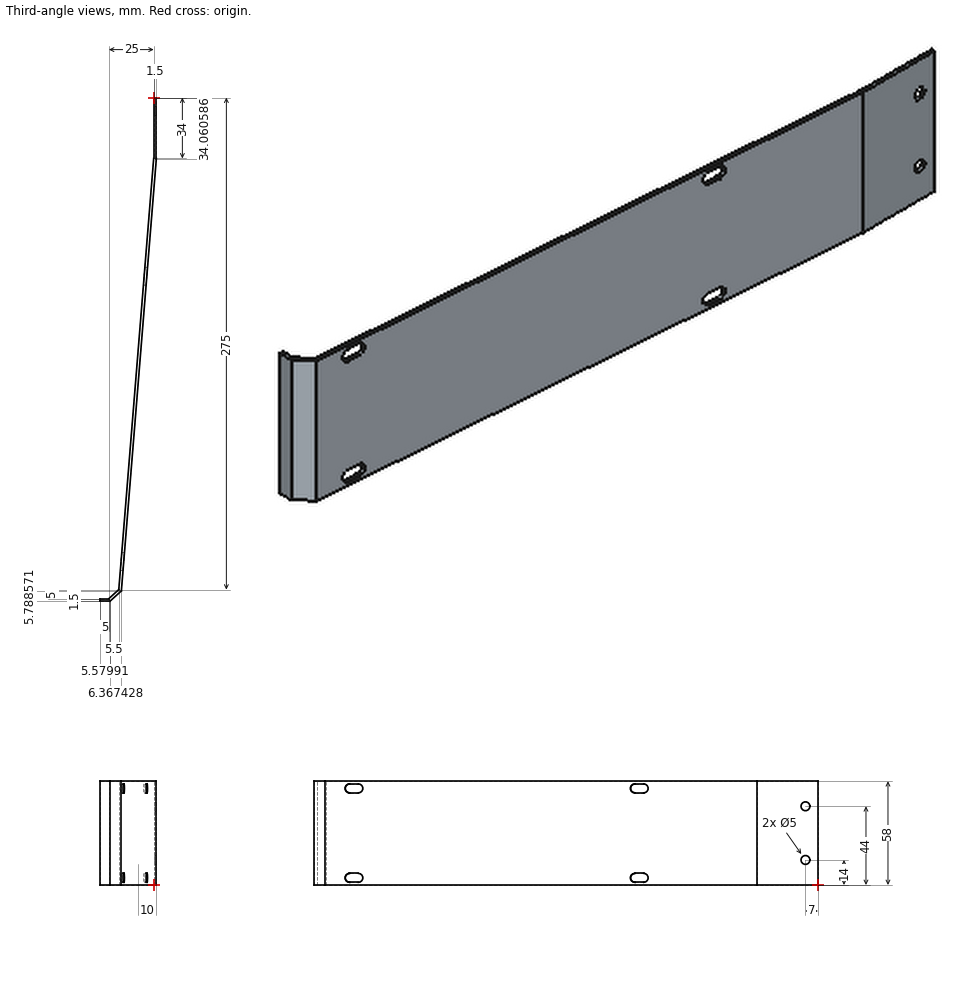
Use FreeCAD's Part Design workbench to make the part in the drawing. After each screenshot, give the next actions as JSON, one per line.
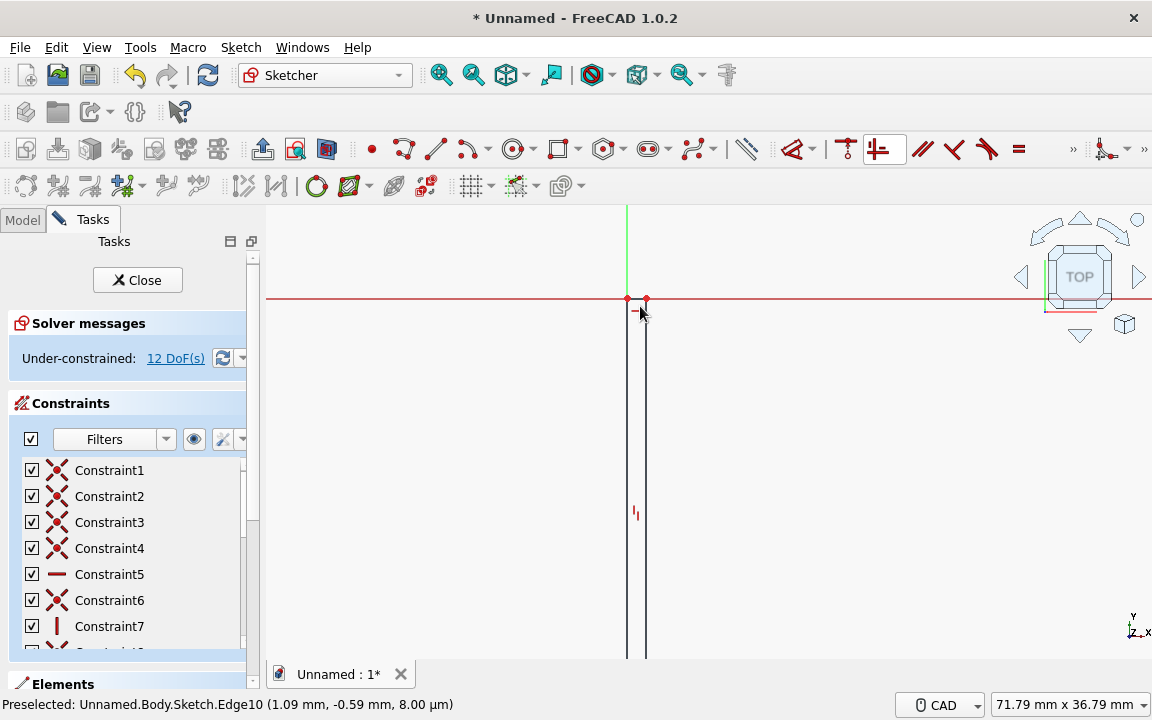
{"action": "left_click", "coordinate": [792, 150]}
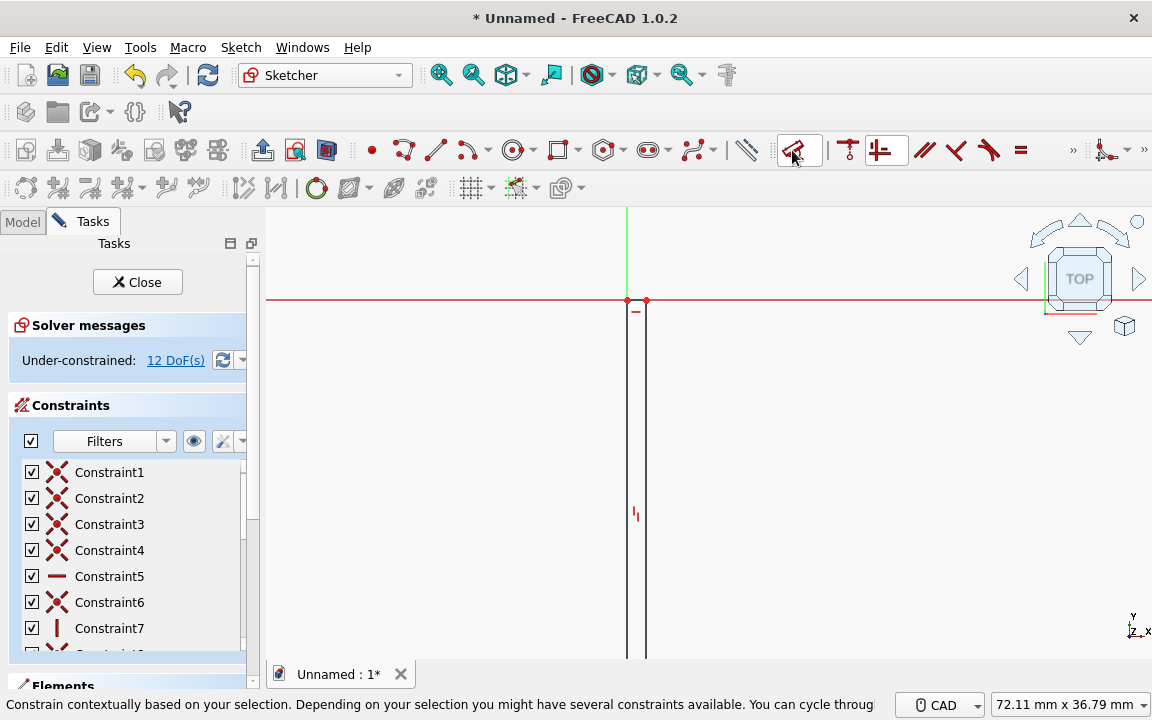
{"action": "scroll", "coordinate": [656, 305], "scroll_direction": "down", "scroll_amount": 13}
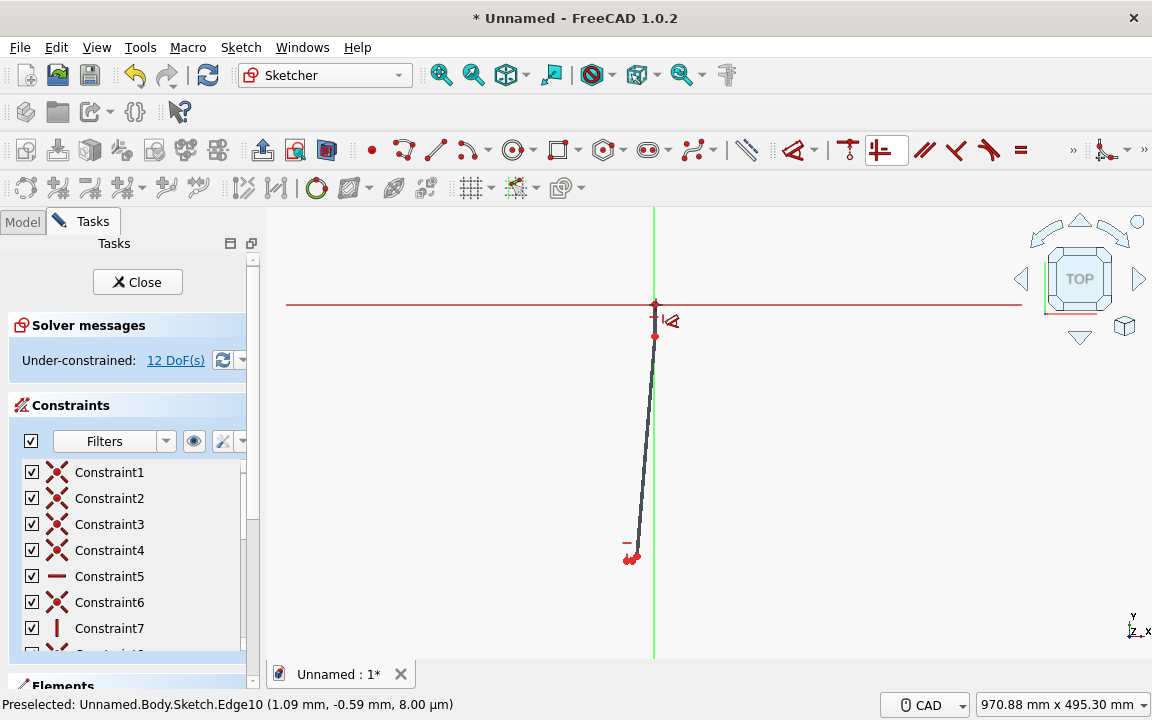
{"action": "scroll", "coordinate": [630, 561], "scroll_direction": "up", "scroll_amount": 13}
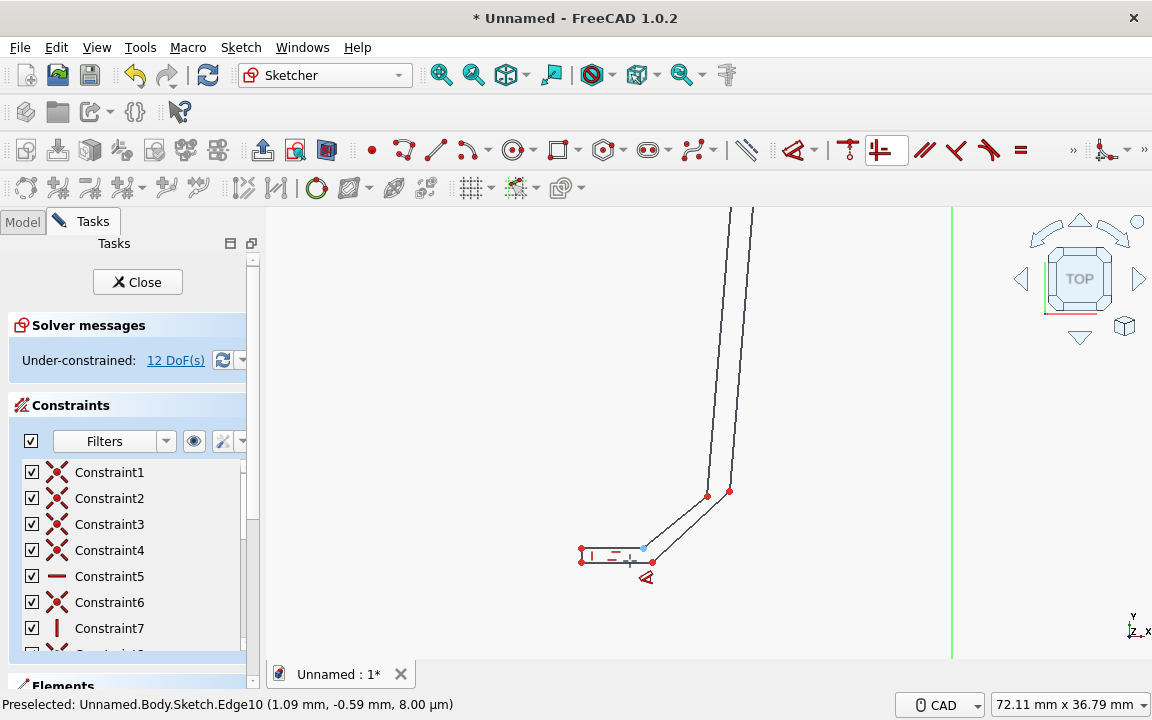
{"action": "left_click", "coordinate": [625, 548]}
{"action": "left_click", "coordinate": [613, 582]}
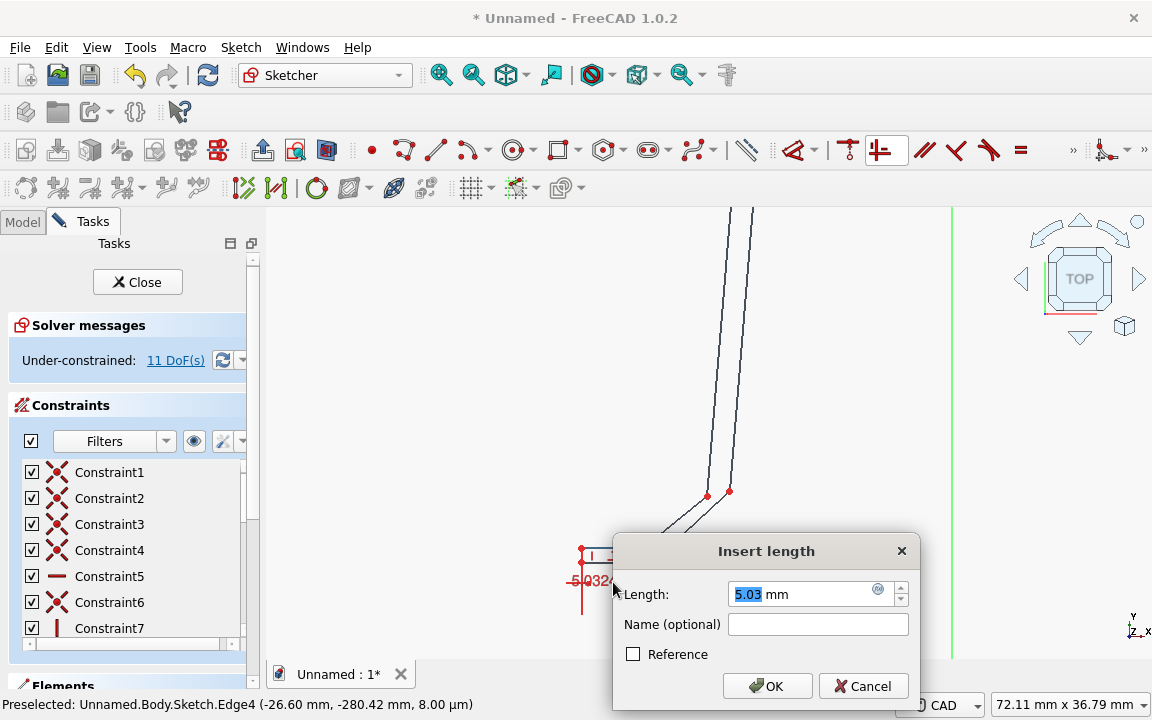
{"action": "type", "text": "5"}
{"action": "key", "text": "Return"}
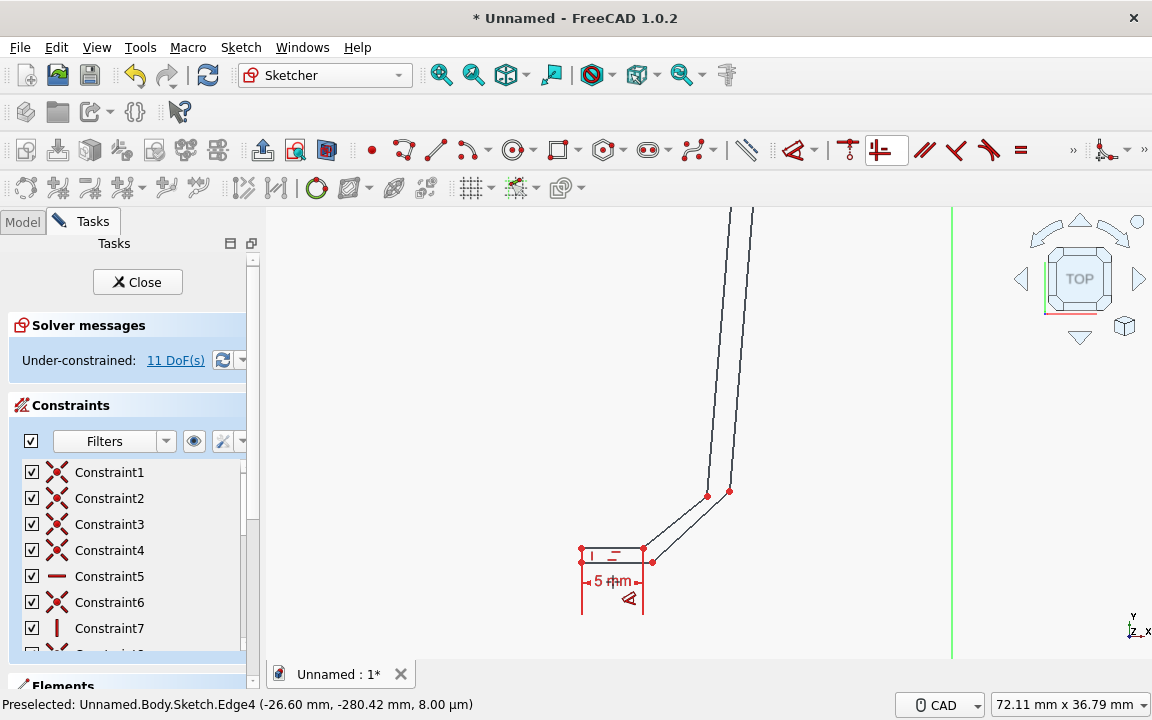
{"action": "scroll", "coordinate": [630, 561], "scroll_direction": "down", "scroll_amount": 13}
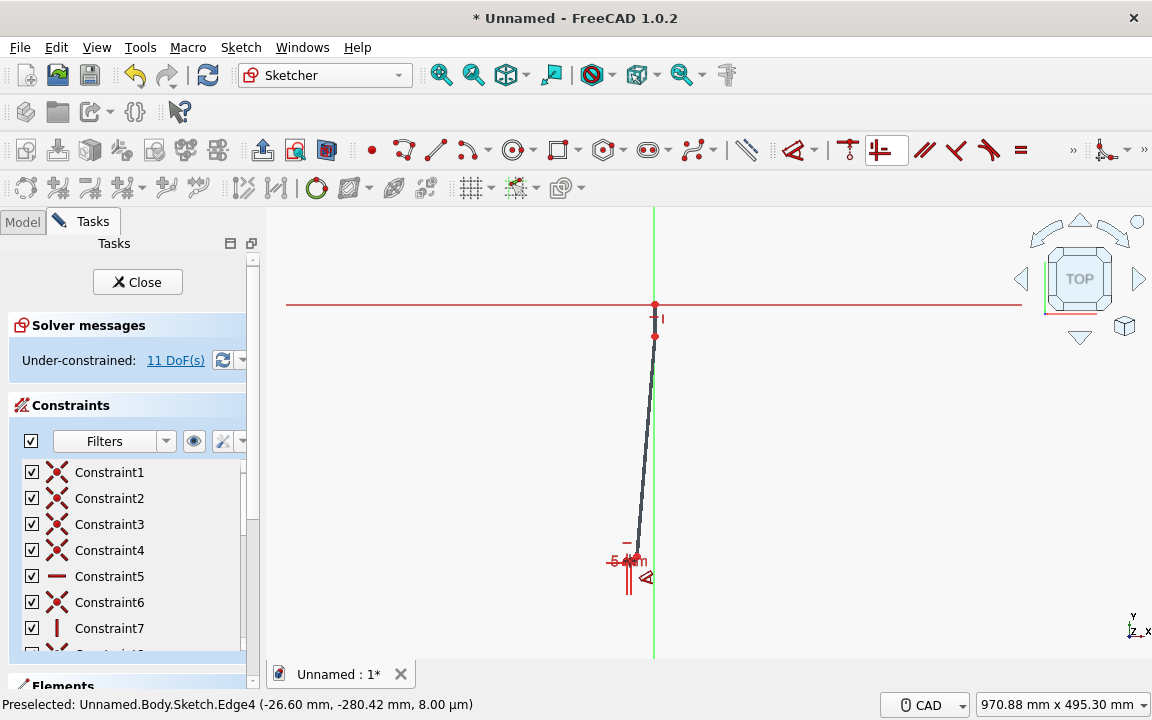
{"action": "scroll", "coordinate": [654, 314], "scroll_direction": "up", "scroll_amount": 12}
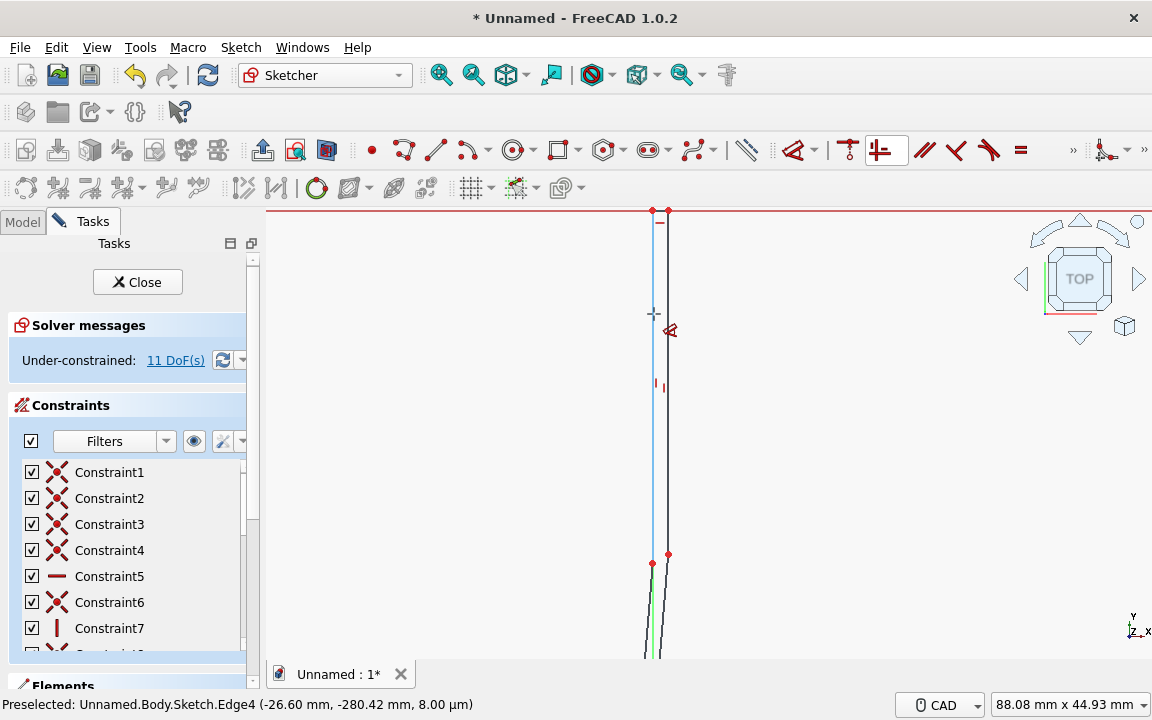
{"action": "left_click", "coordinate": [653, 317]}
{"action": "left_click", "coordinate": [687, 399]}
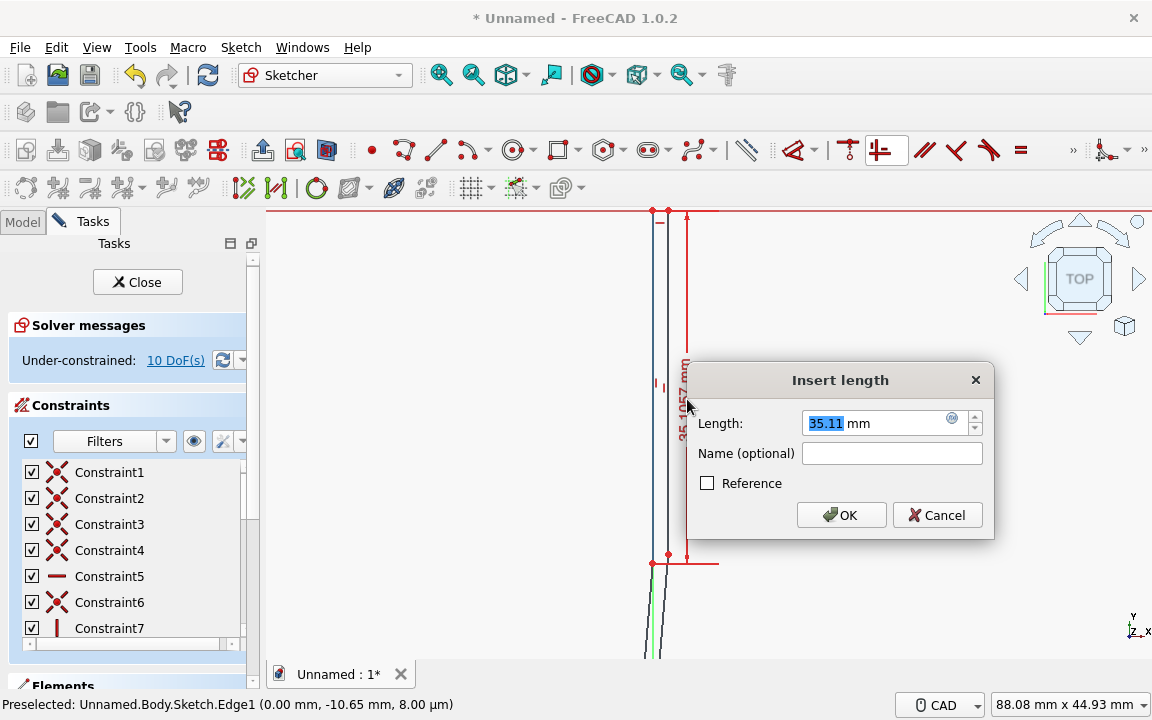
{"action": "type", "text": "34"}
{"action": "key", "text": "Return"}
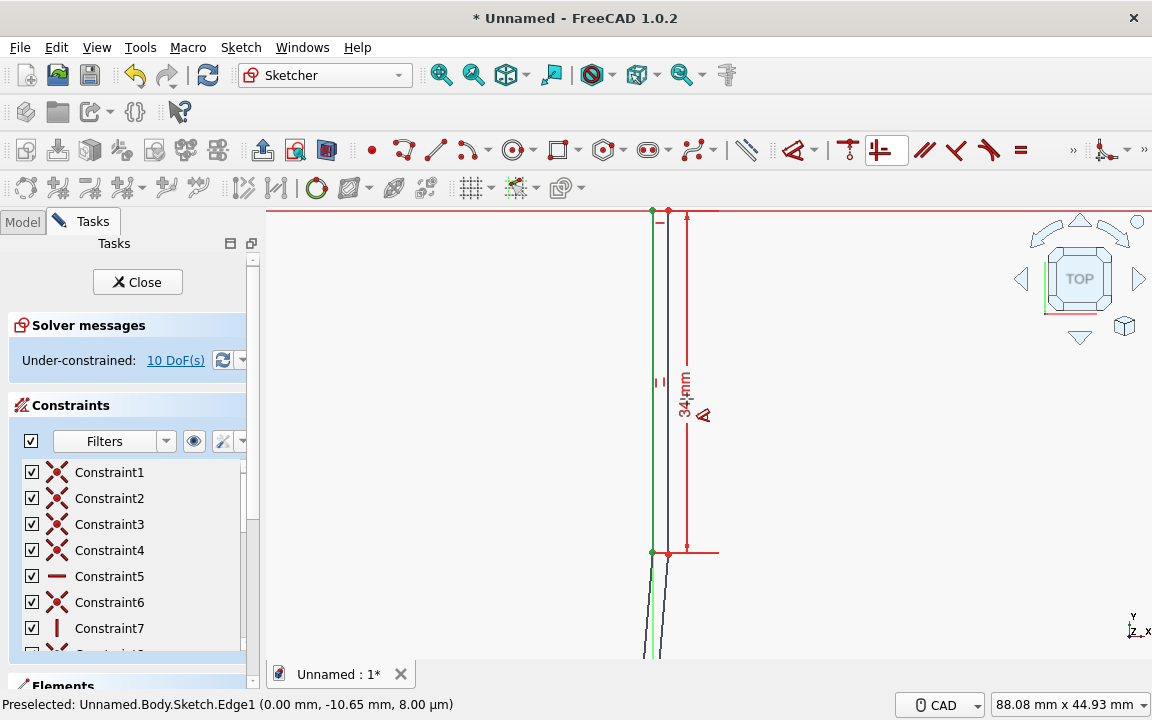
{"action": "scroll", "coordinate": [654, 314], "scroll_direction": "down", "scroll_amount": 12}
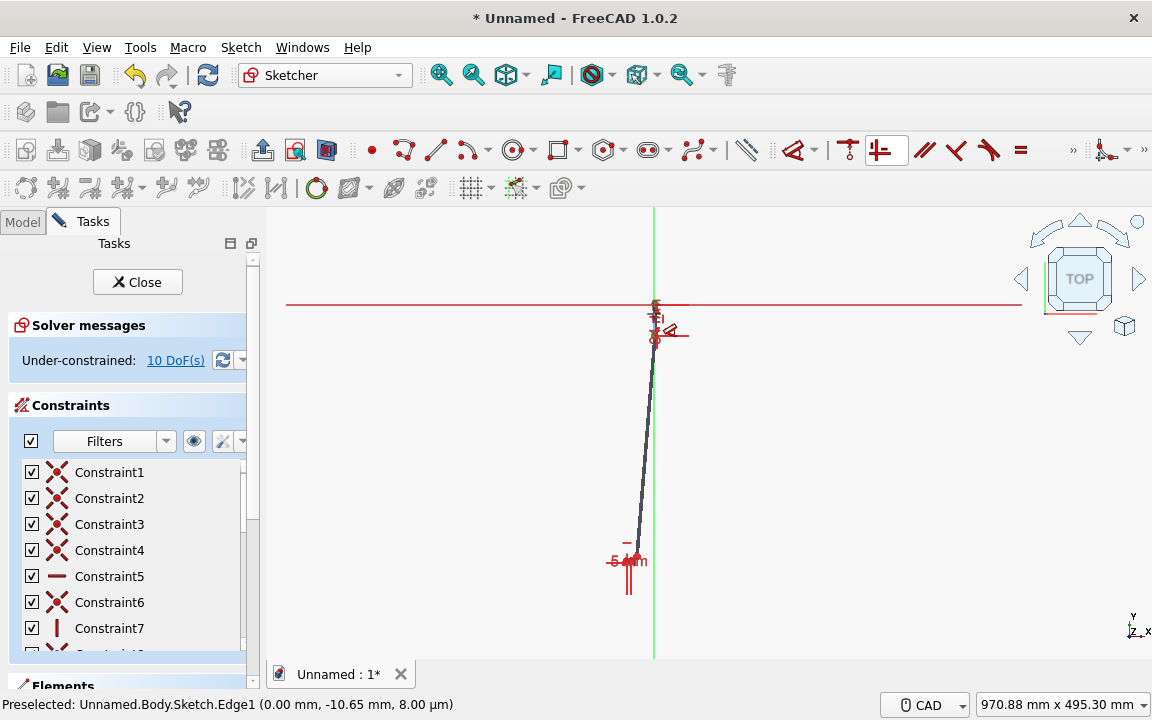
{"action": "scroll", "coordinate": [635, 558], "scroll_direction": "up", "scroll_amount": 14}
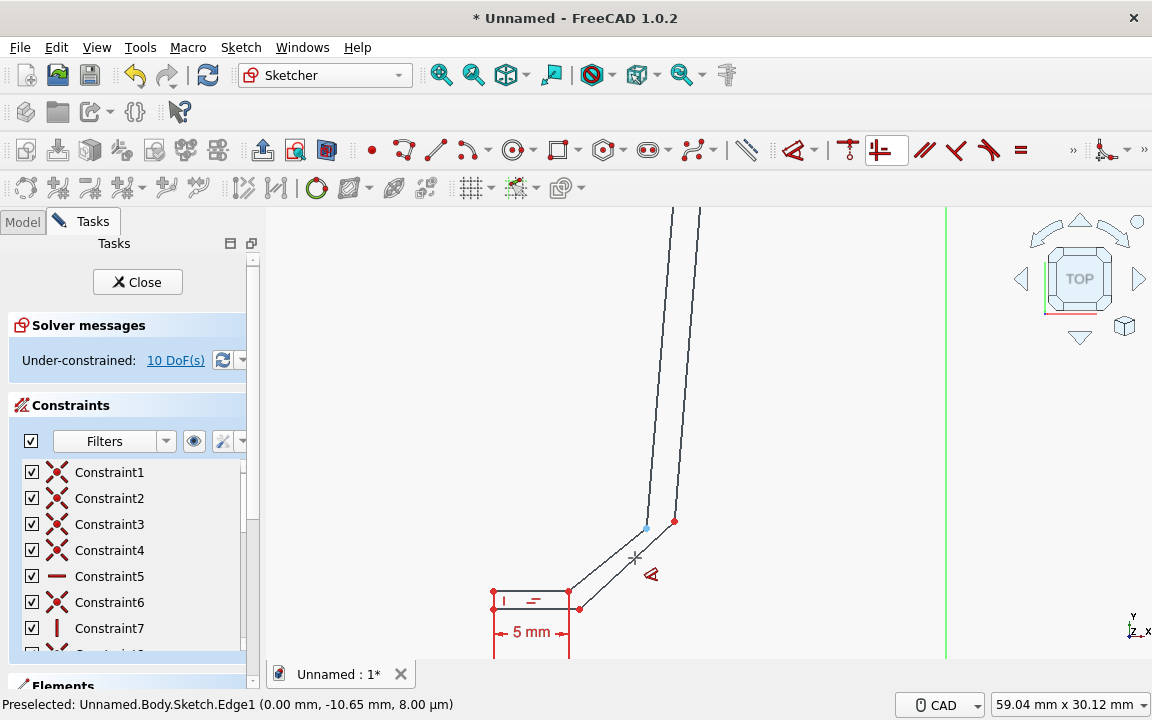
{"action": "left_click", "coordinate": [623, 547]}
{"action": "left_click", "coordinate": [535, 560]}